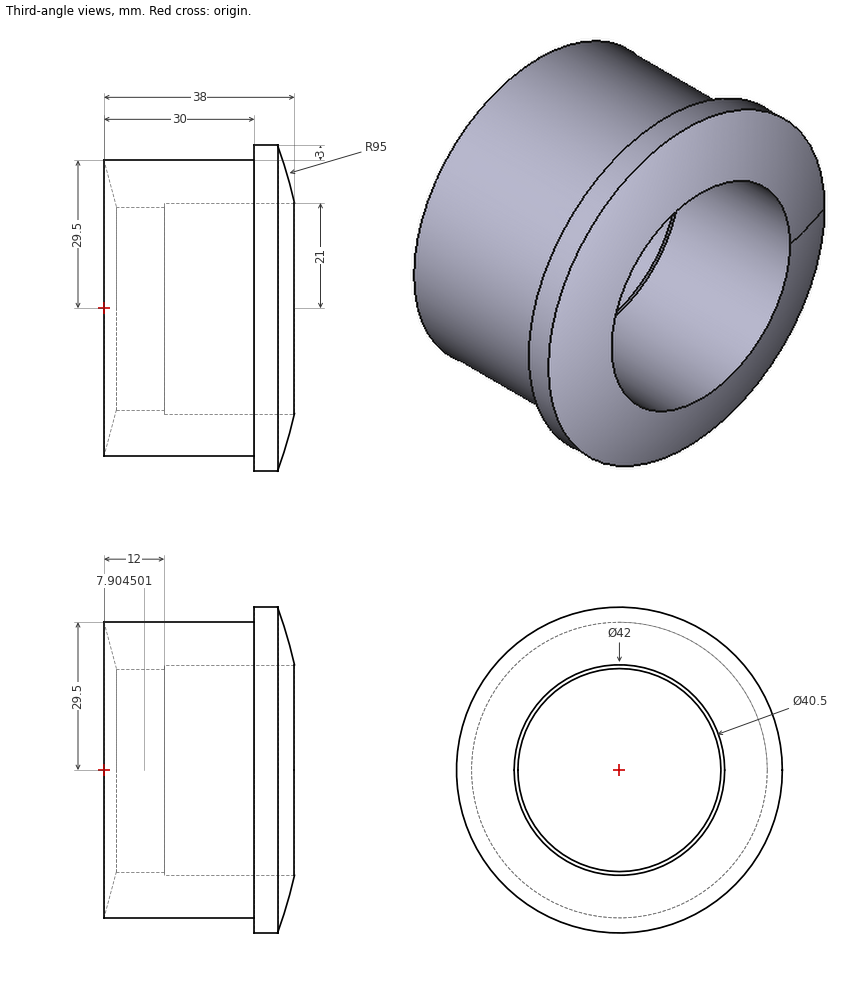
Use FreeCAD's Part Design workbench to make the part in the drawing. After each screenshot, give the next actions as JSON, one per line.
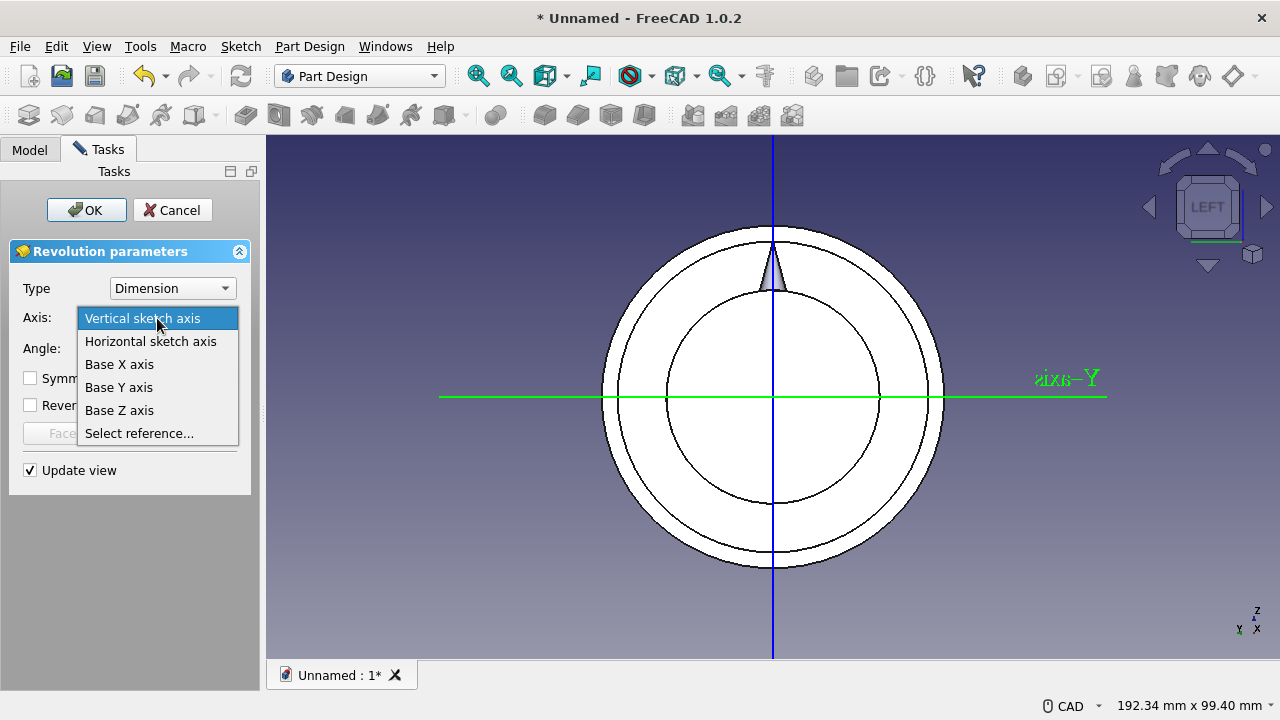
{"action": "left_click", "coordinate": [156, 342]}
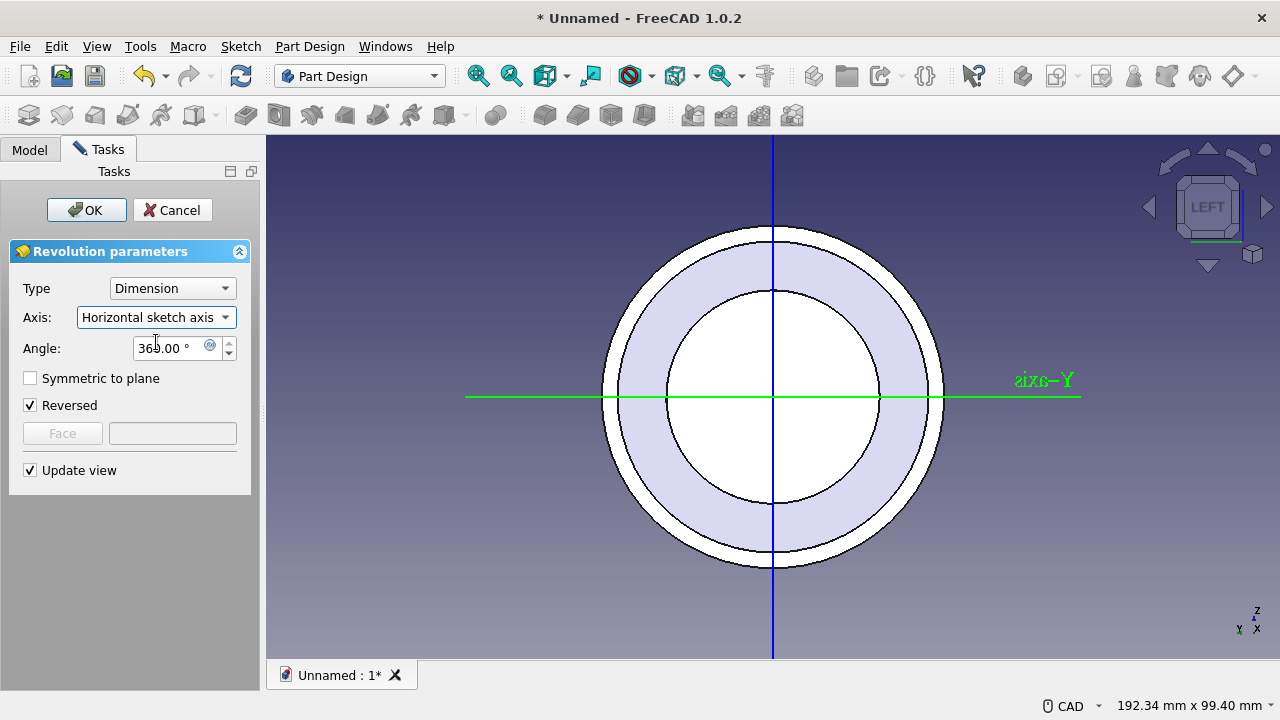
{"action": "left_click", "coordinate": [87, 210]}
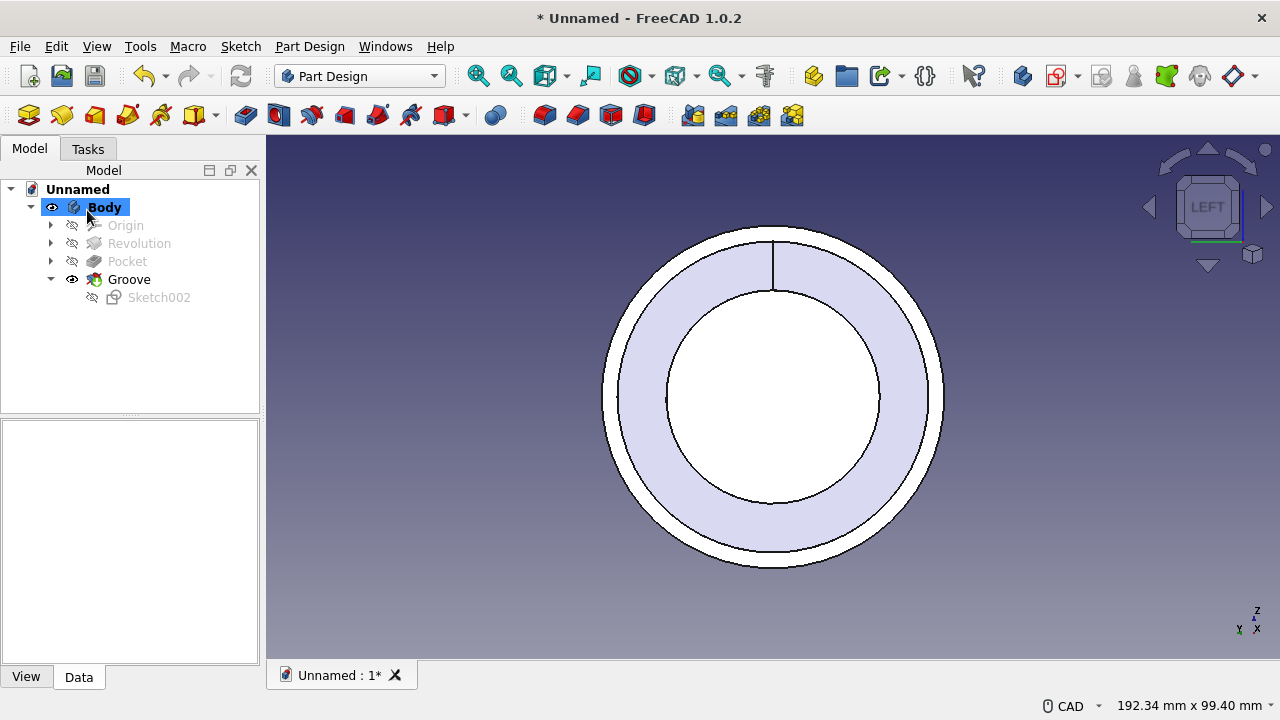
{"action": "left_click", "coordinate": [773, 396]}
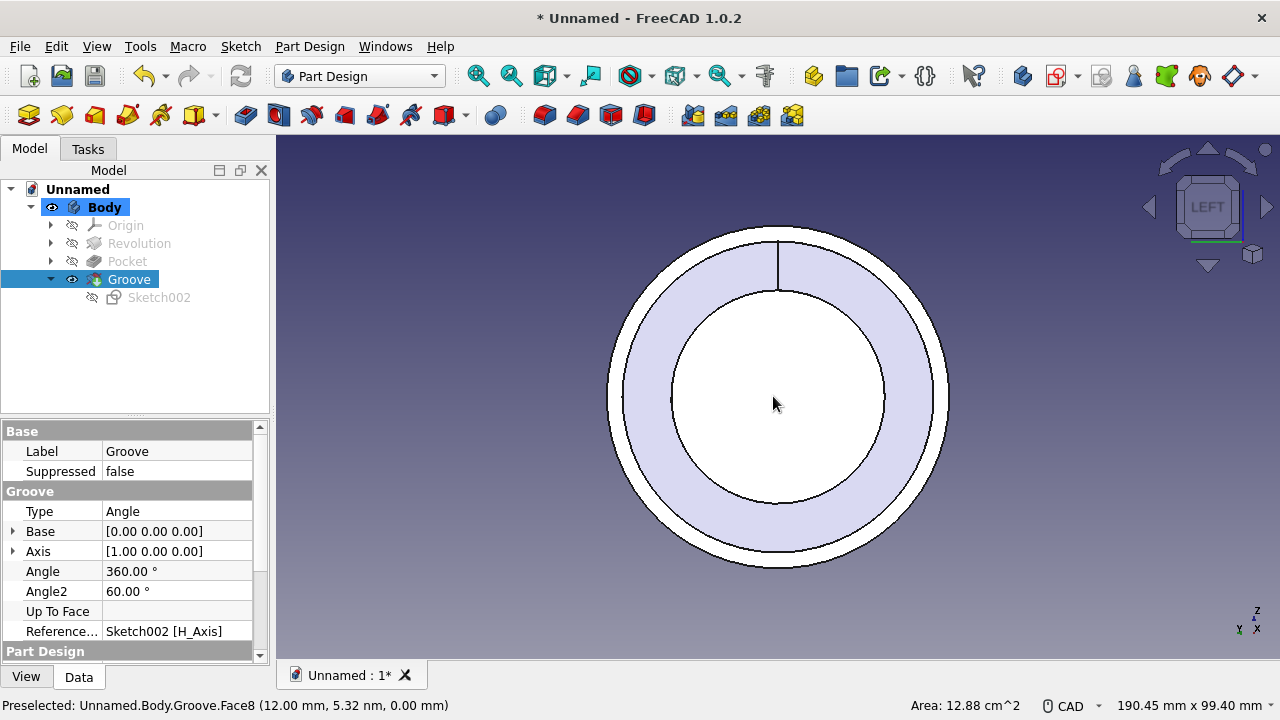
{"action": "left_click", "coordinate": [1056, 76]}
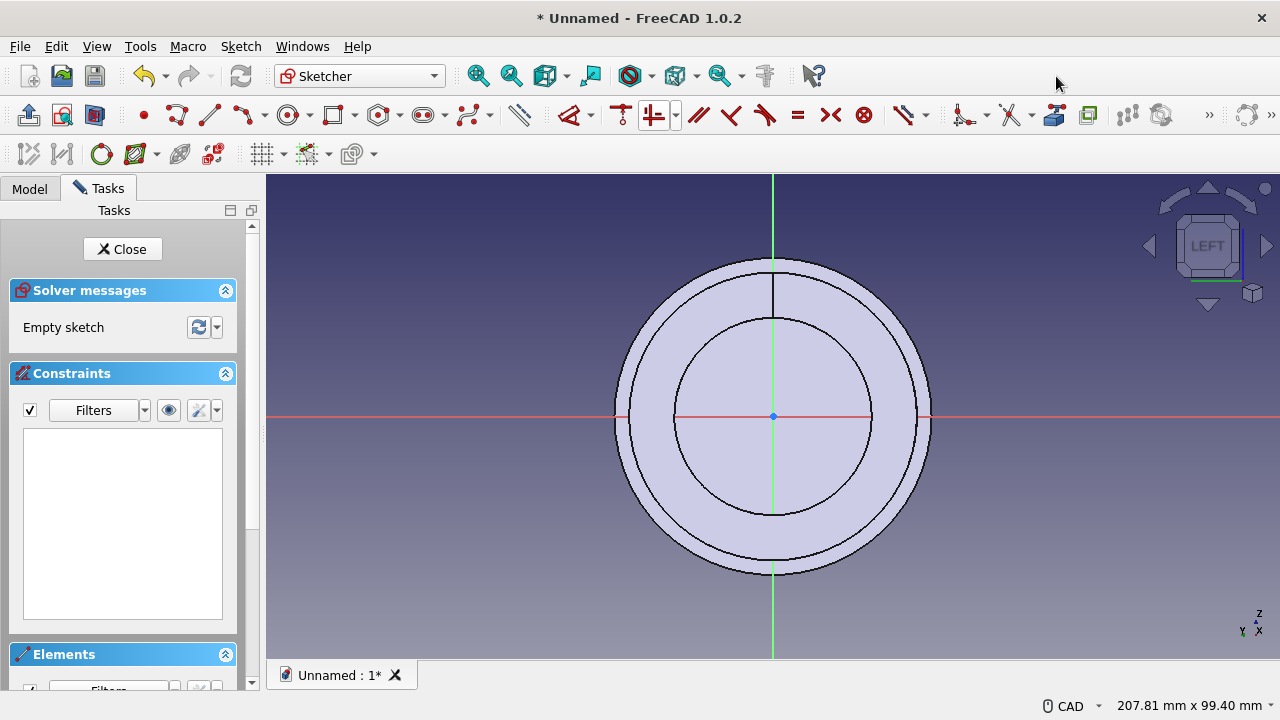
{"action": "left_click", "coordinate": [95, 116]}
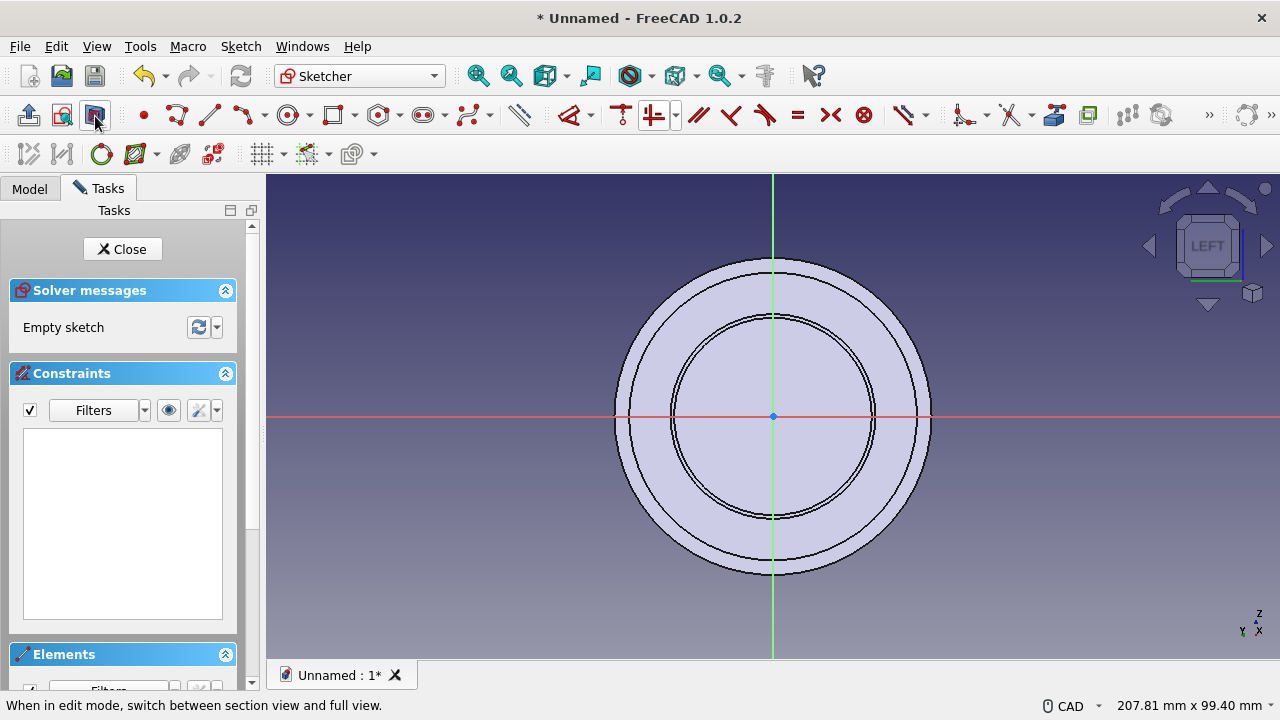
{"action": "scroll", "coordinate": [912, 417], "scroll_direction": "up", "scroll_amount": 2}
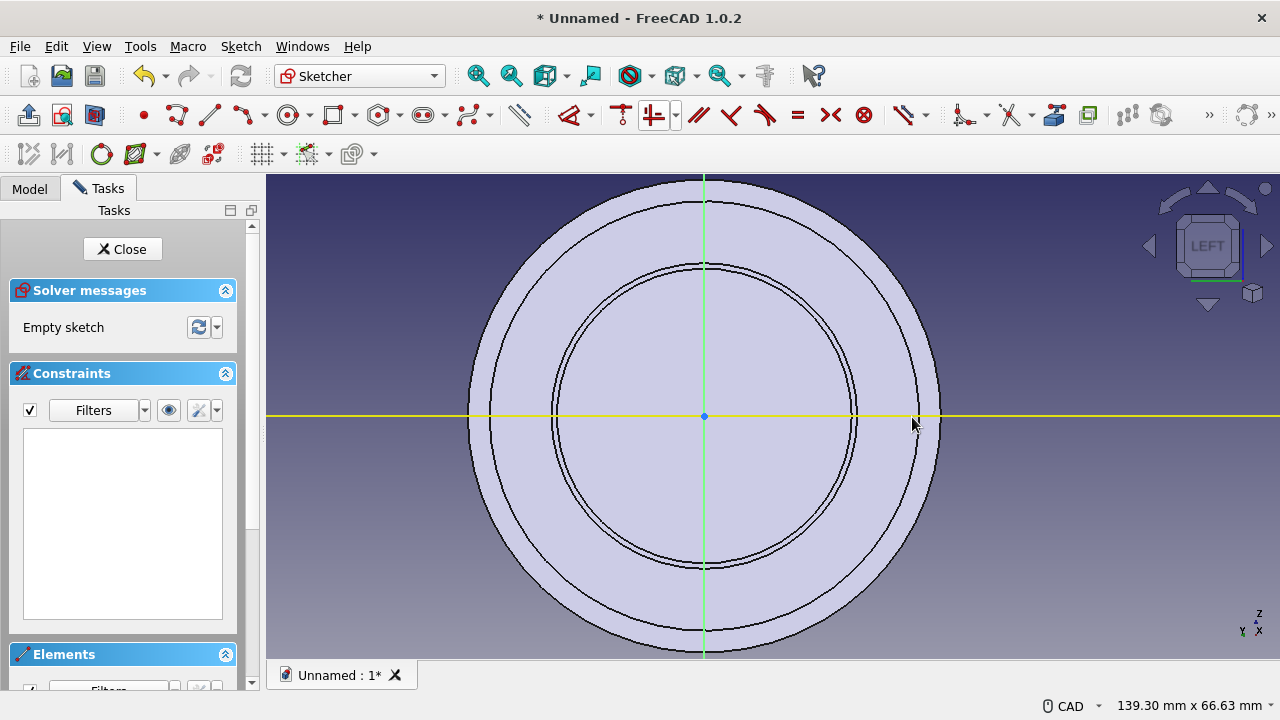
{"action": "left_click", "coordinate": [288, 116]}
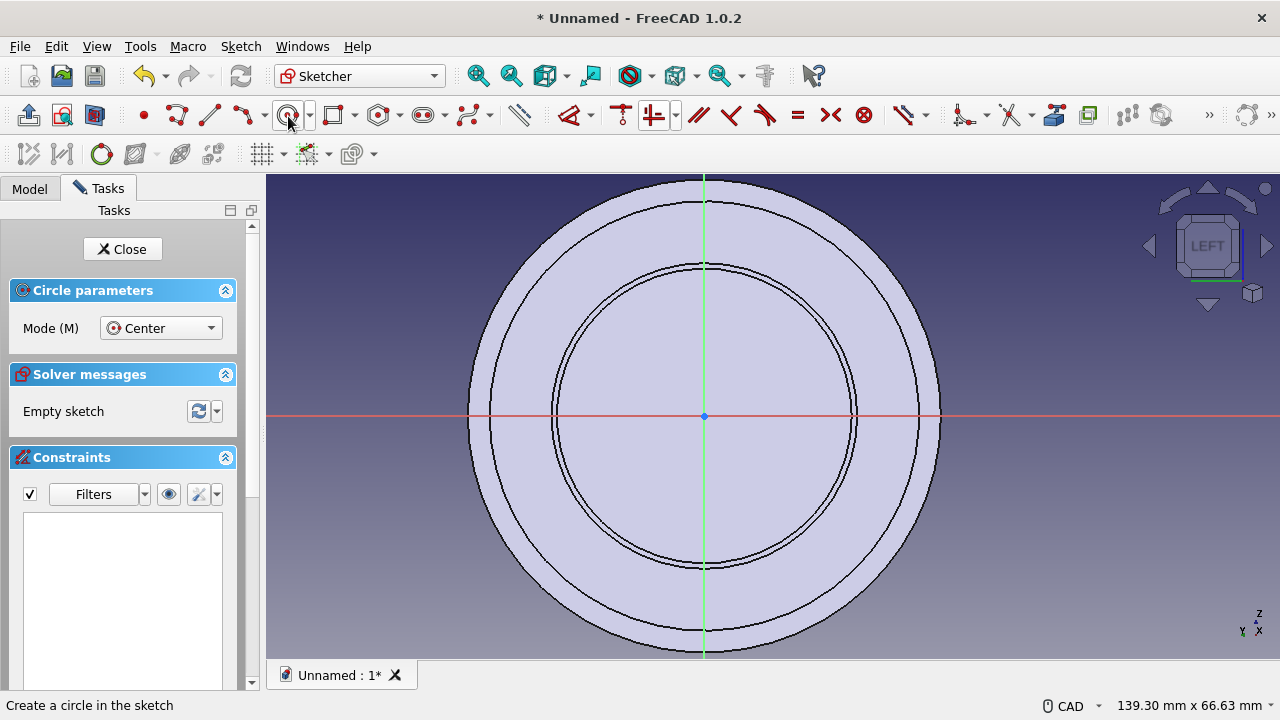
{"action": "left_click", "coordinate": [704, 416]}
{"action": "mouse_move", "coordinate": [812, 308]}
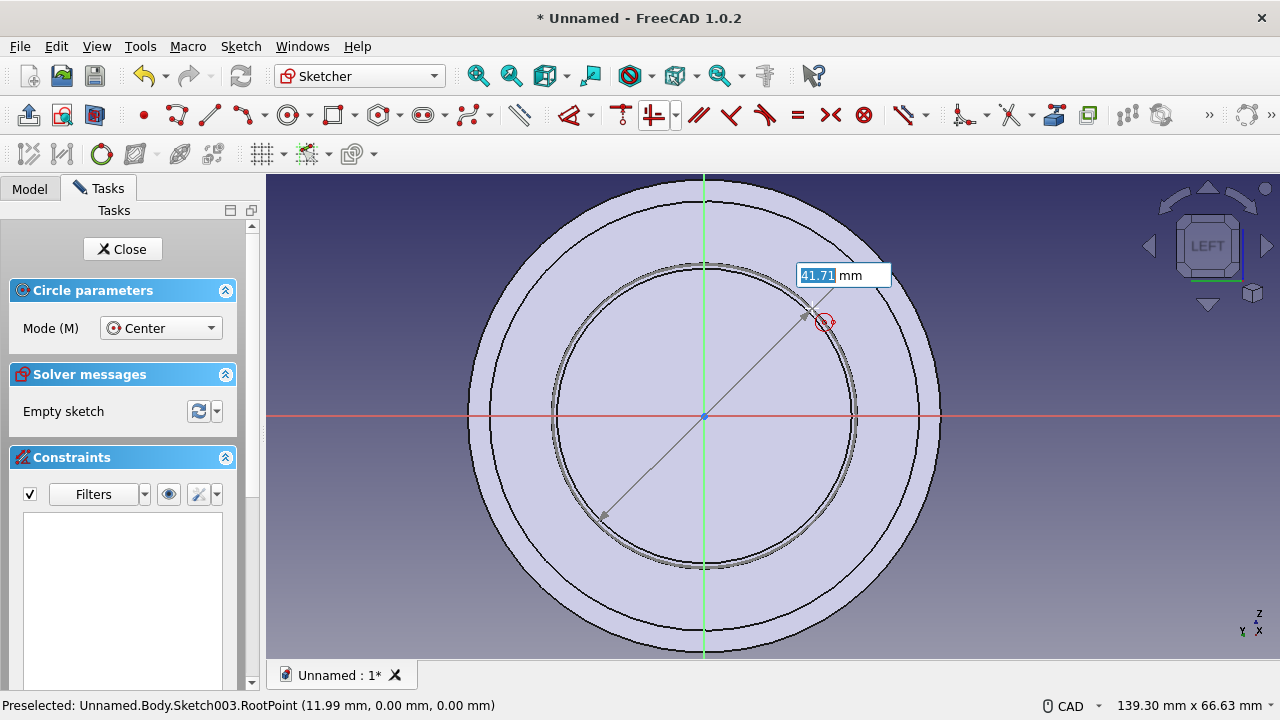
{"action": "type", "text": "42"}
{"action": "key", "text": "Return"}
{"action": "key", "text": "Escape"}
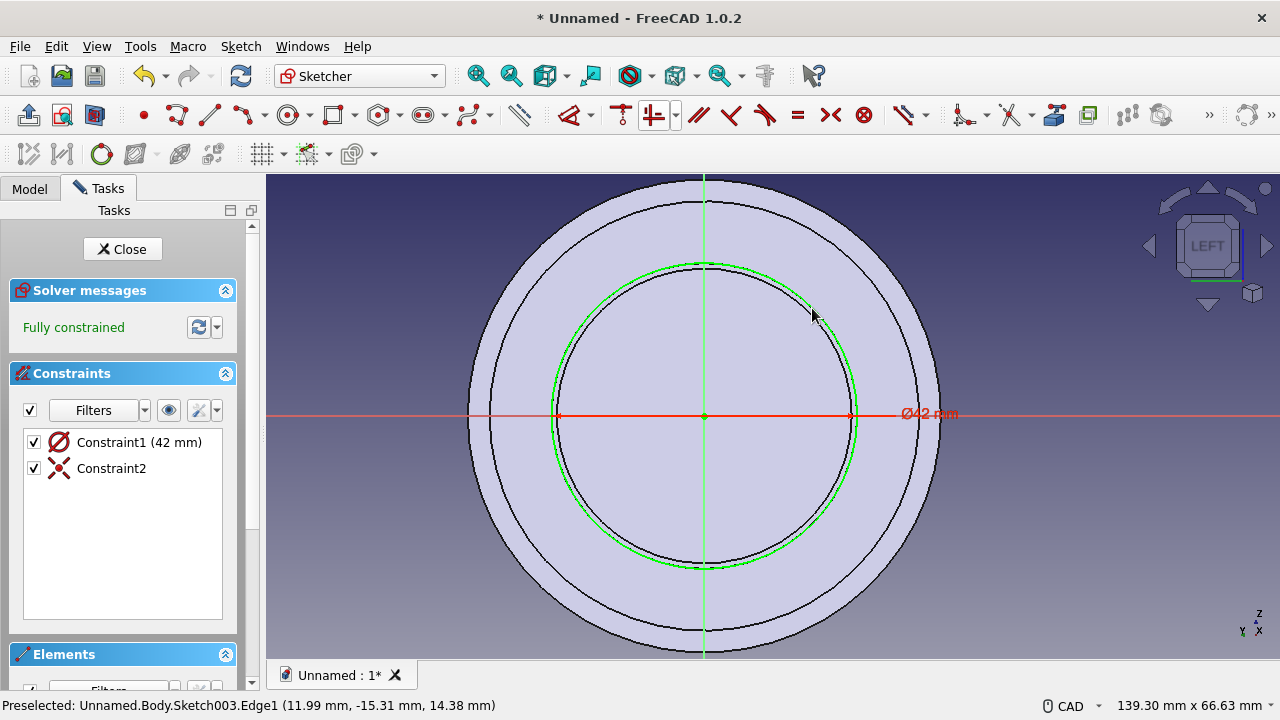
{"action": "left_click", "coordinate": [123, 249]}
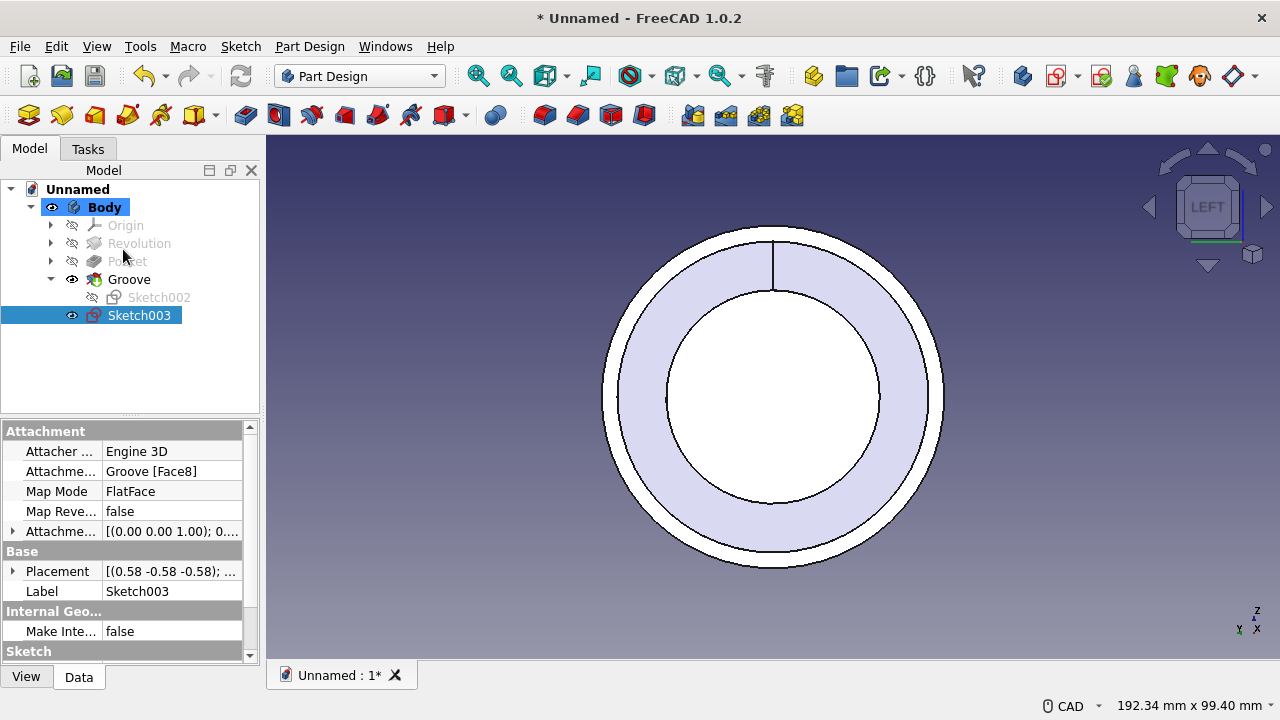
{"action": "left_click", "coordinate": [246, 116]}